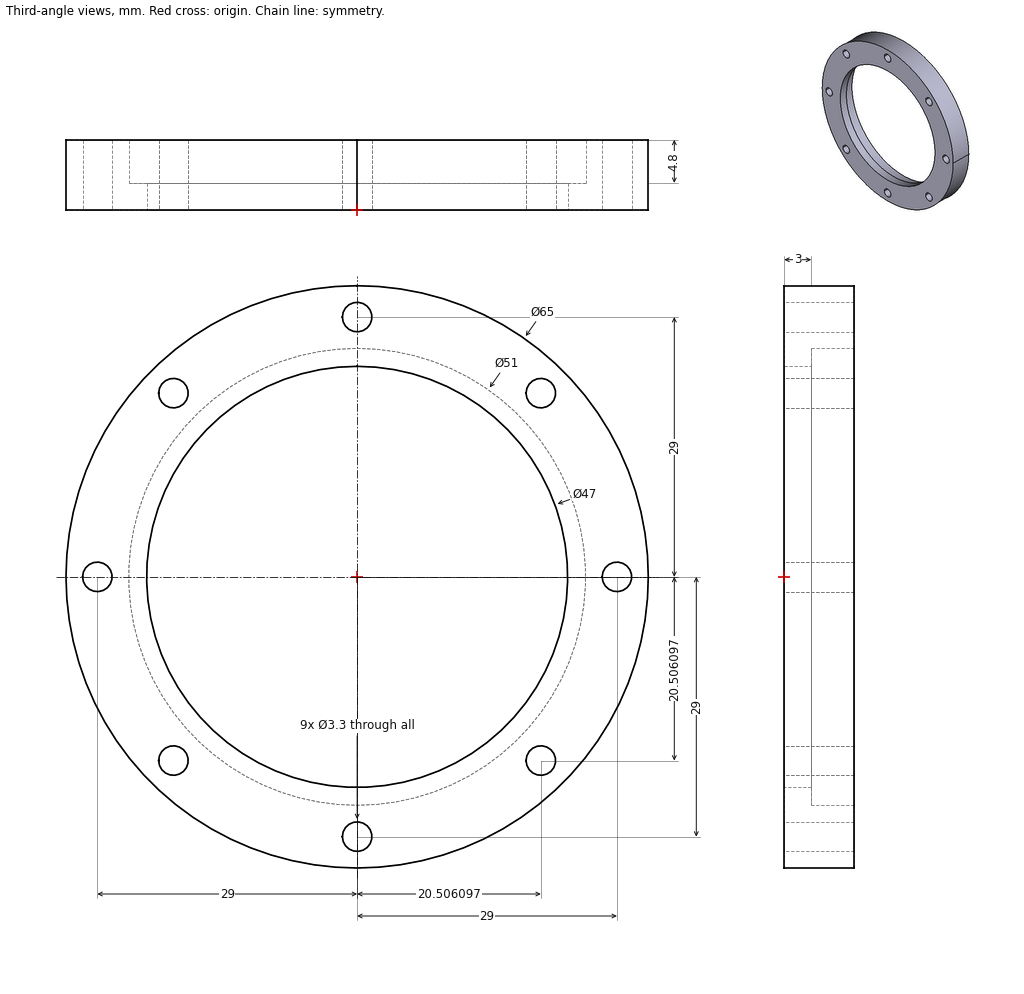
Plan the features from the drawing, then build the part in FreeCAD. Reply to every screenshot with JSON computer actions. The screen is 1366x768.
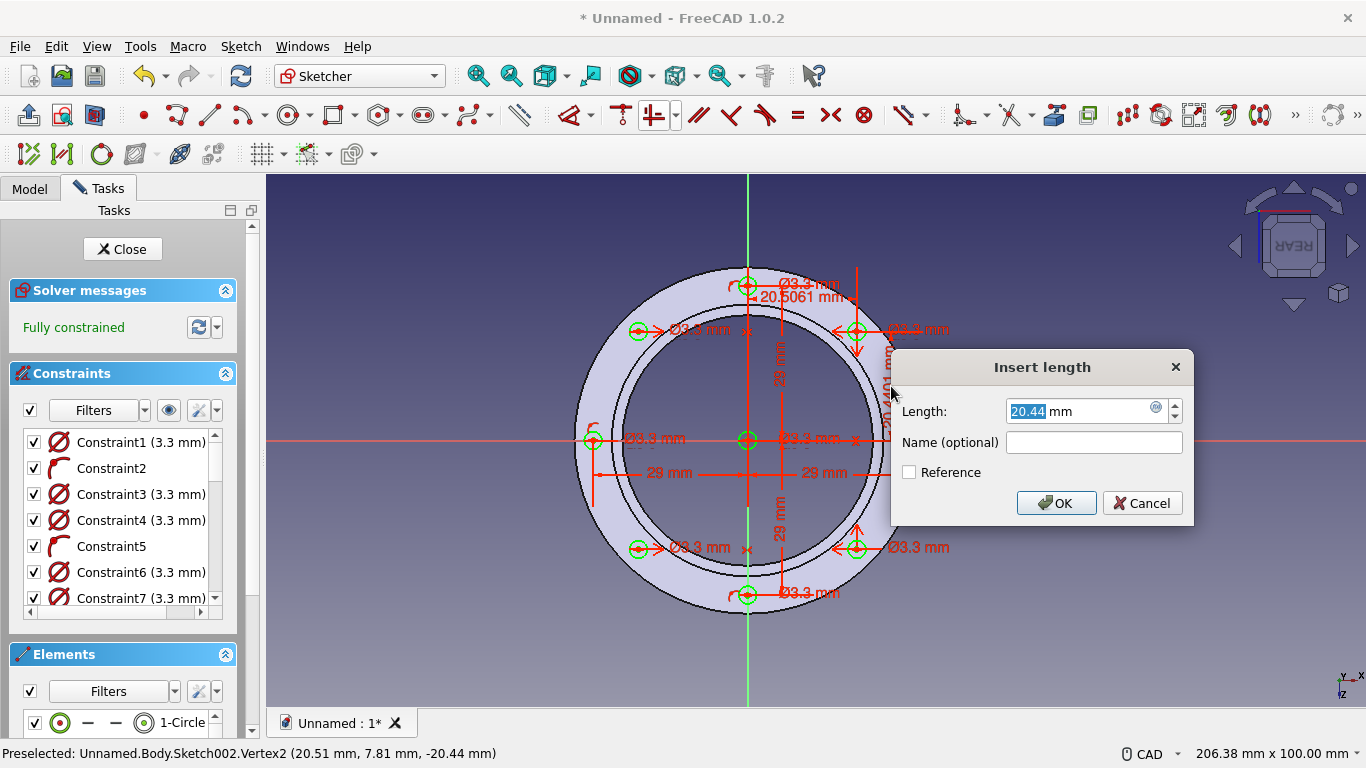
{"action": "type", "text": "20.506097"}
{"action": "key", "text": "Return"}
{"action": "key", "text": "Escape"}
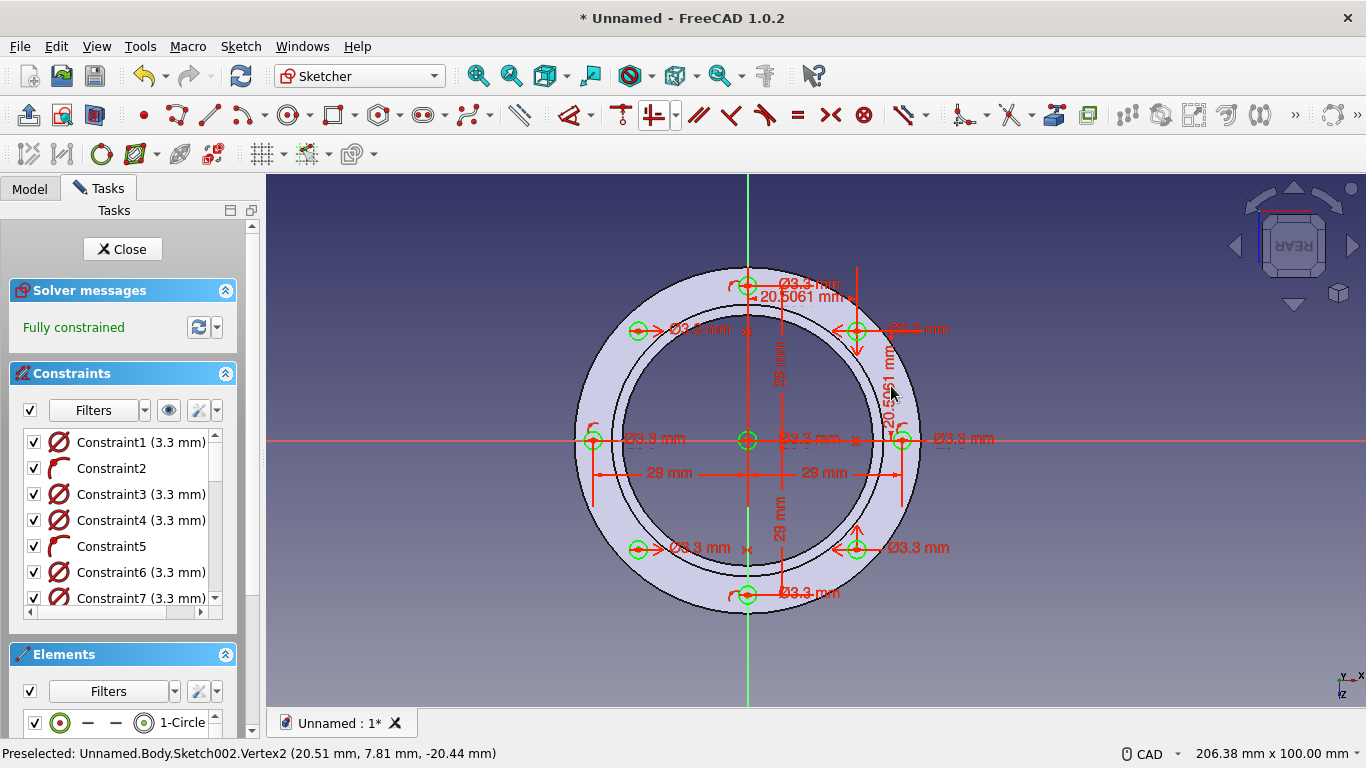
{"action": "left_click", "coordinate": [123, 249]}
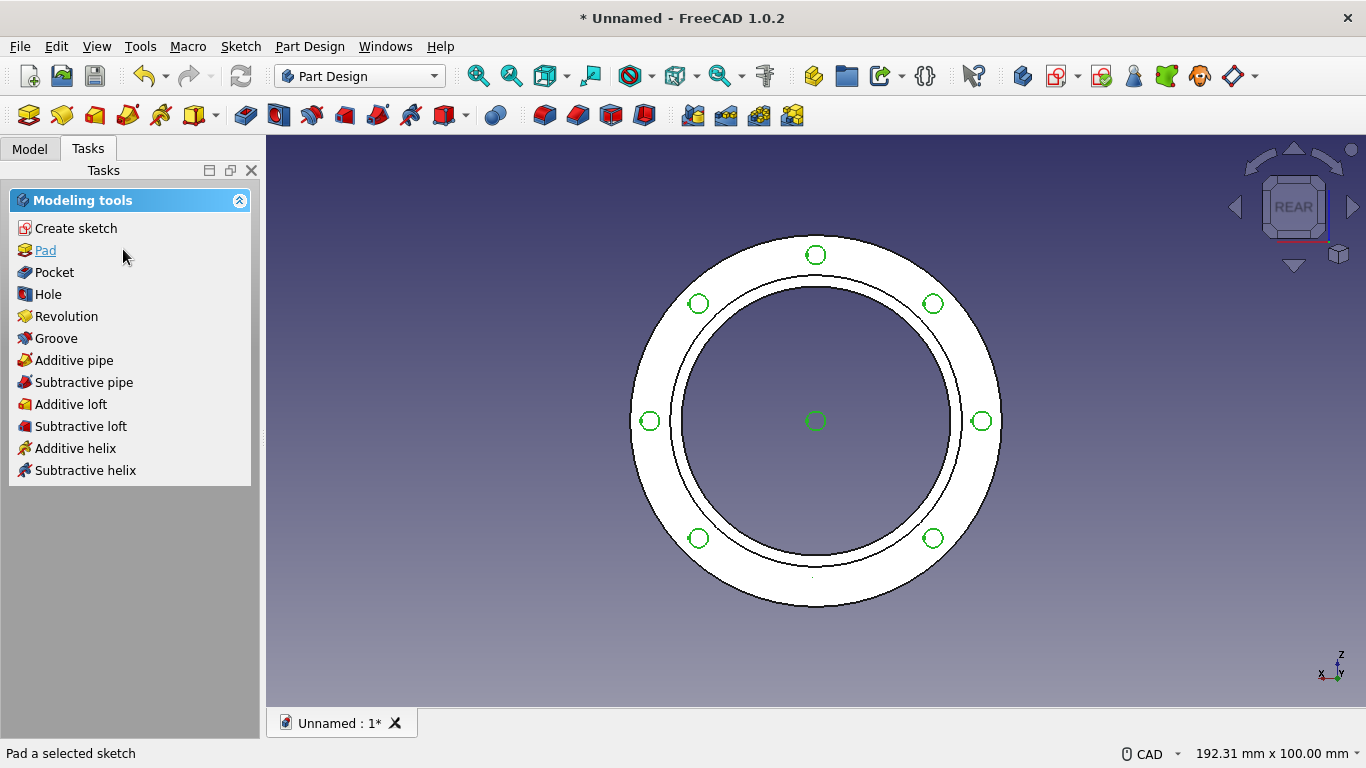
{"action": "left_click", "coordinate": [279, 116]}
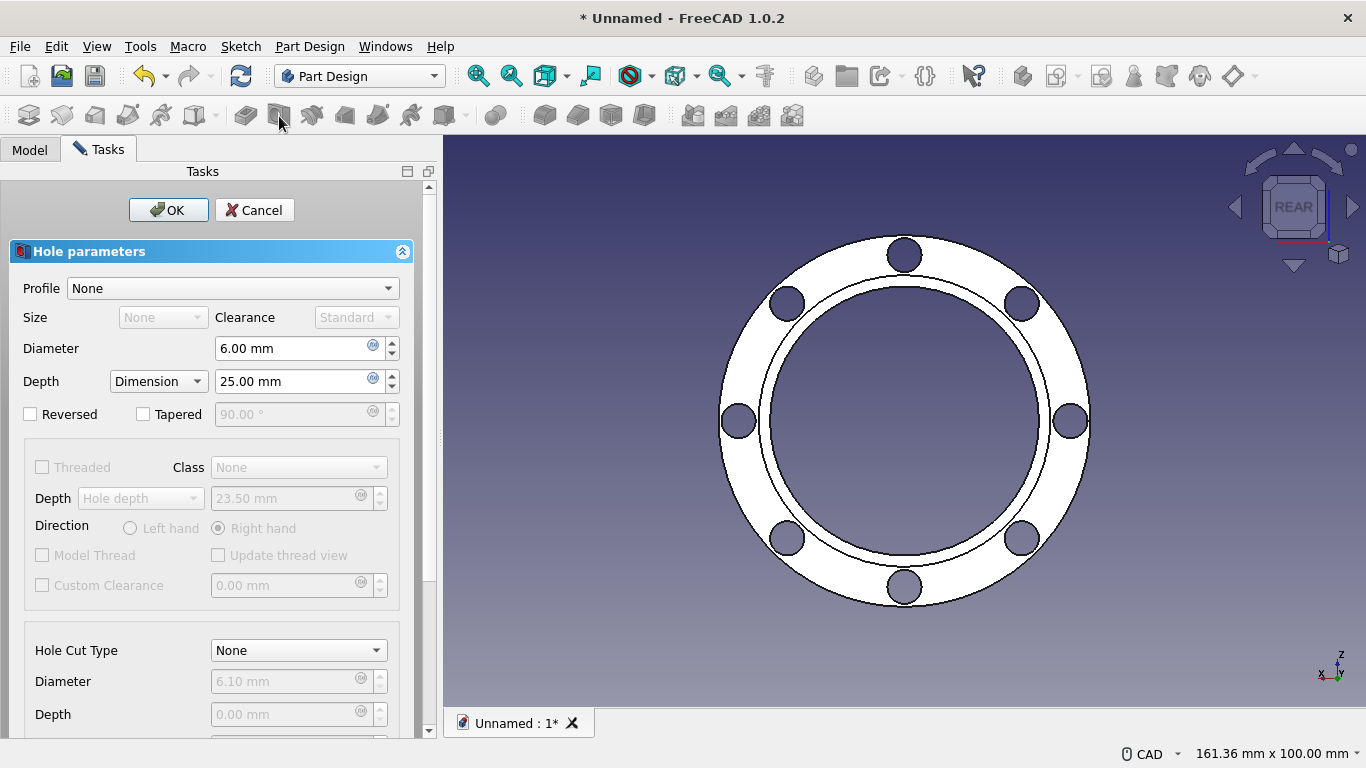
{"action": "triple_click", "coordinate": [300, 348]}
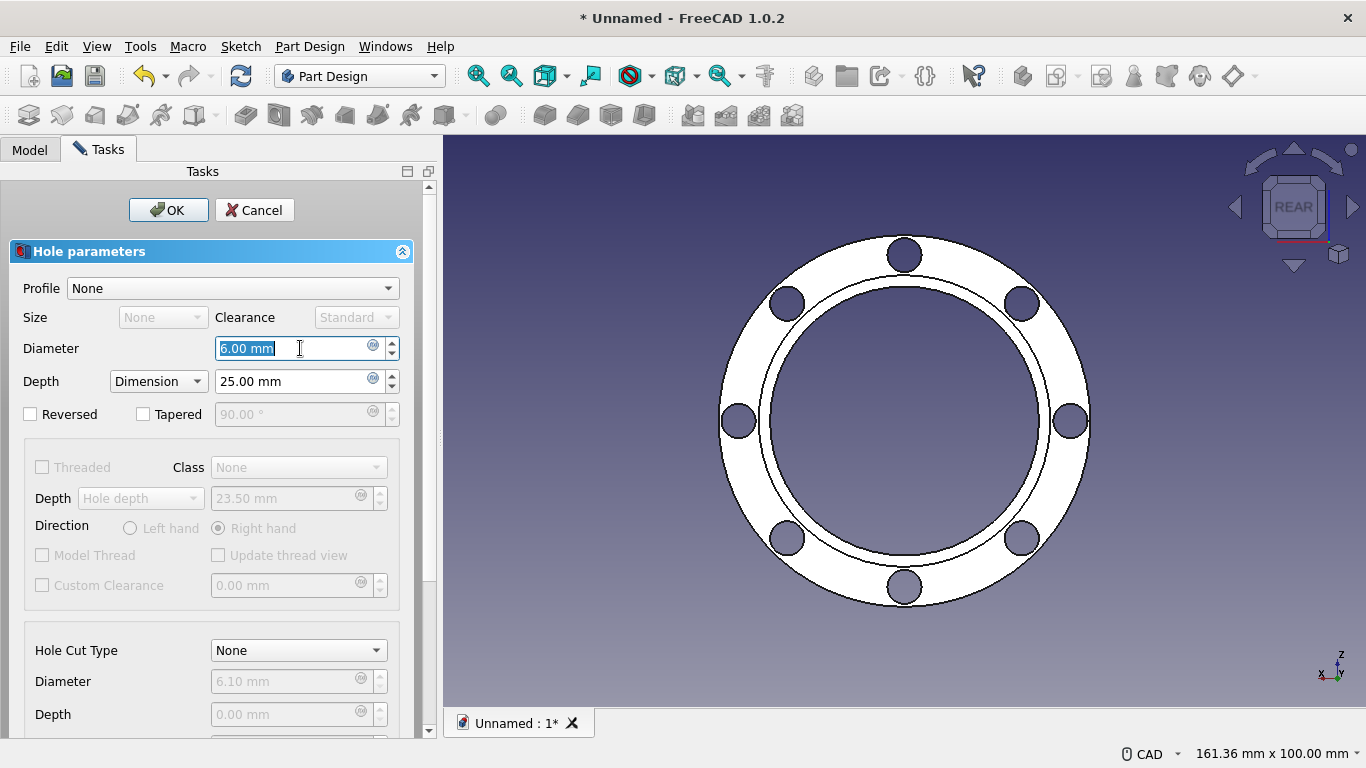
{"action": "type", "text": "3.3"}
{"action": "key", "text": "Tab"}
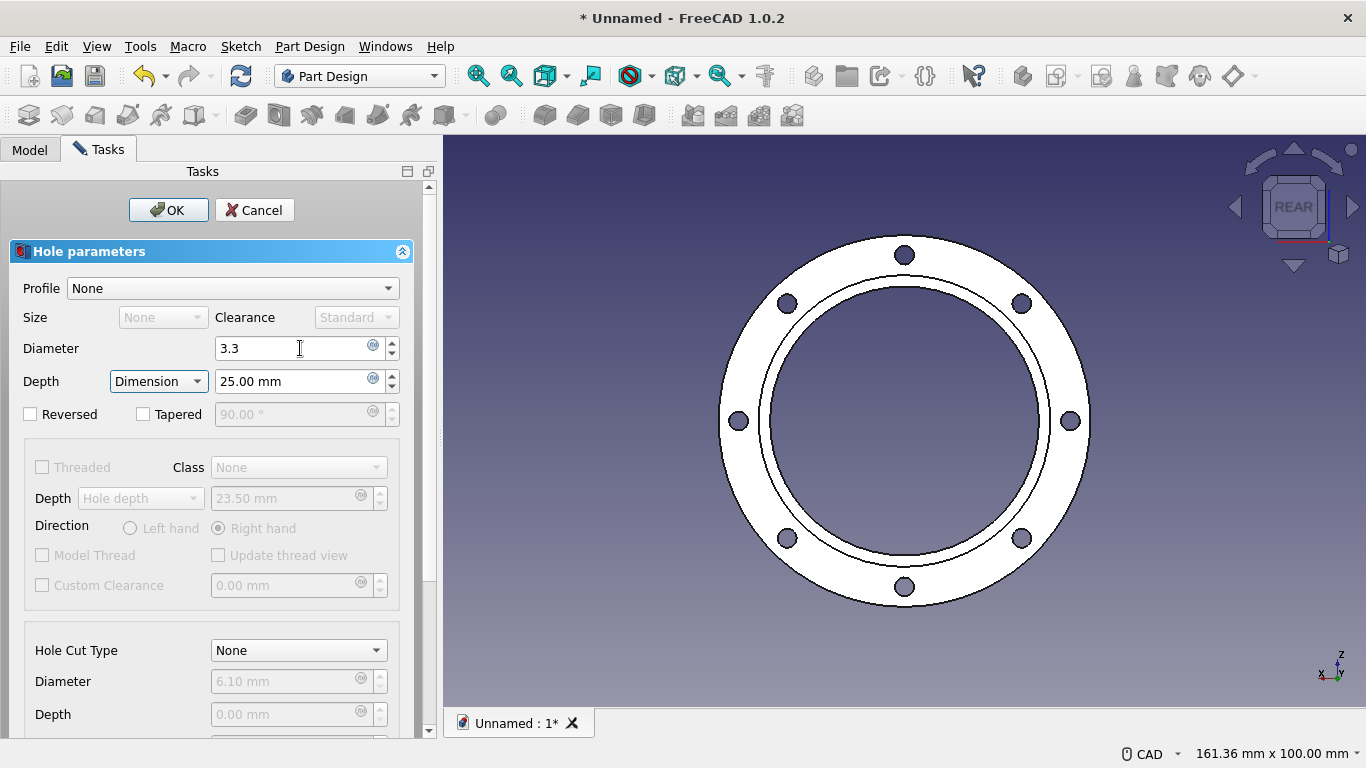
{"action": "left_click", "coordinate": [160, 382]}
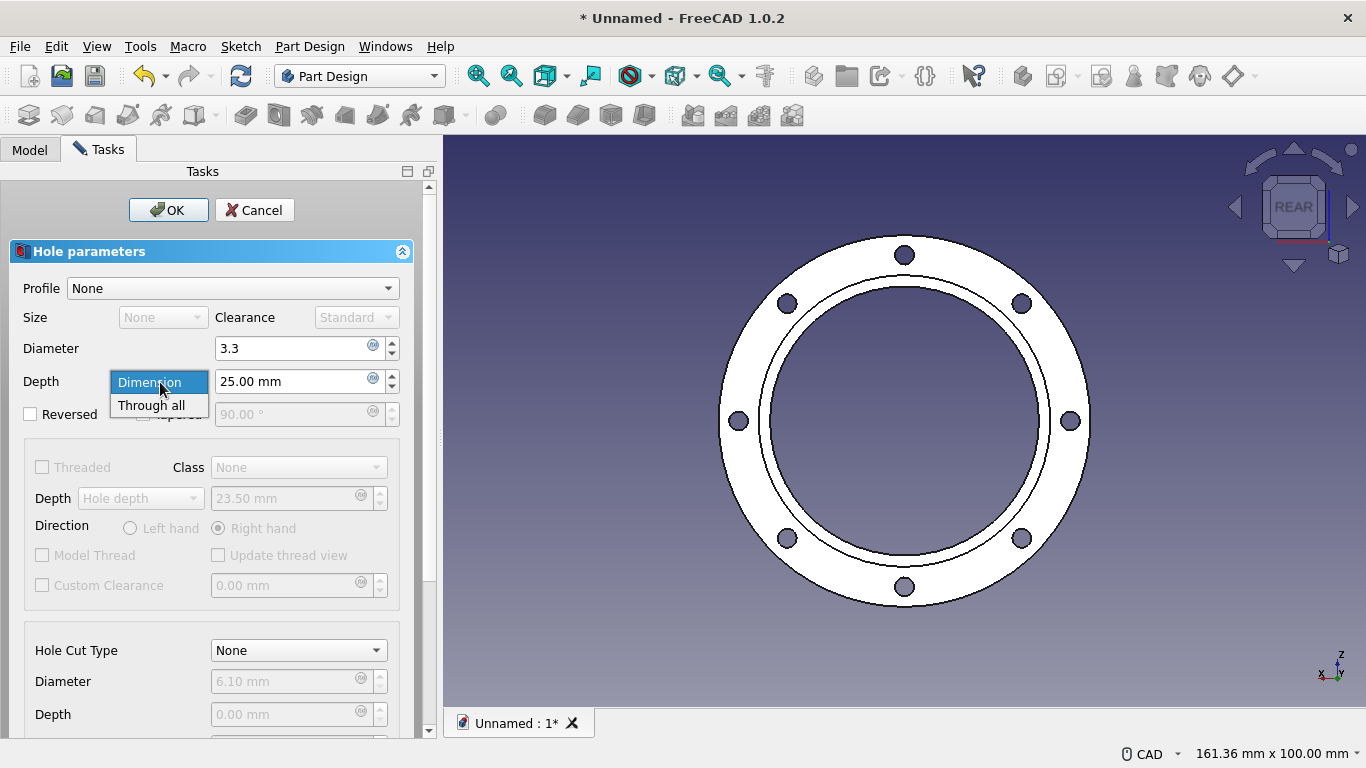
{"action": "left_click", "coordinate": [158, 406]}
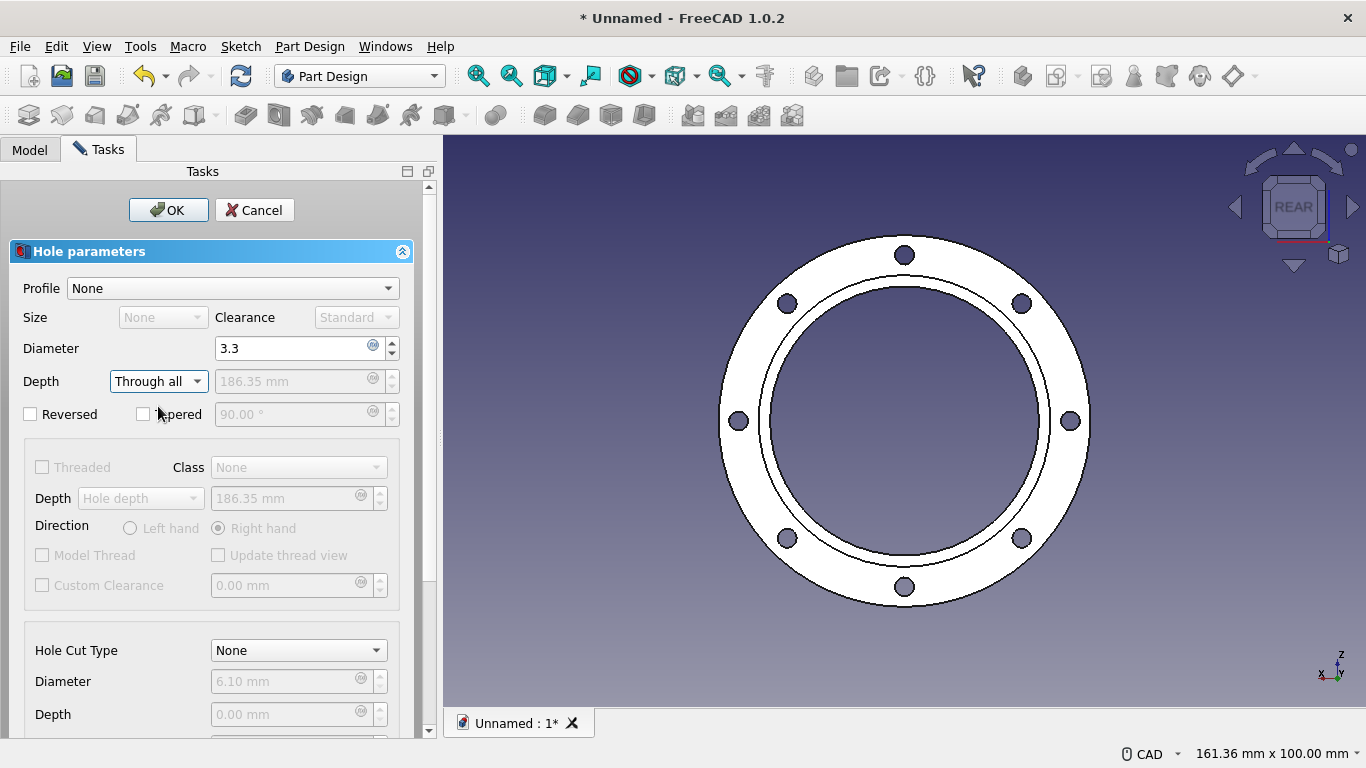
{"action": "left_click", "coordinate": [169, 210]}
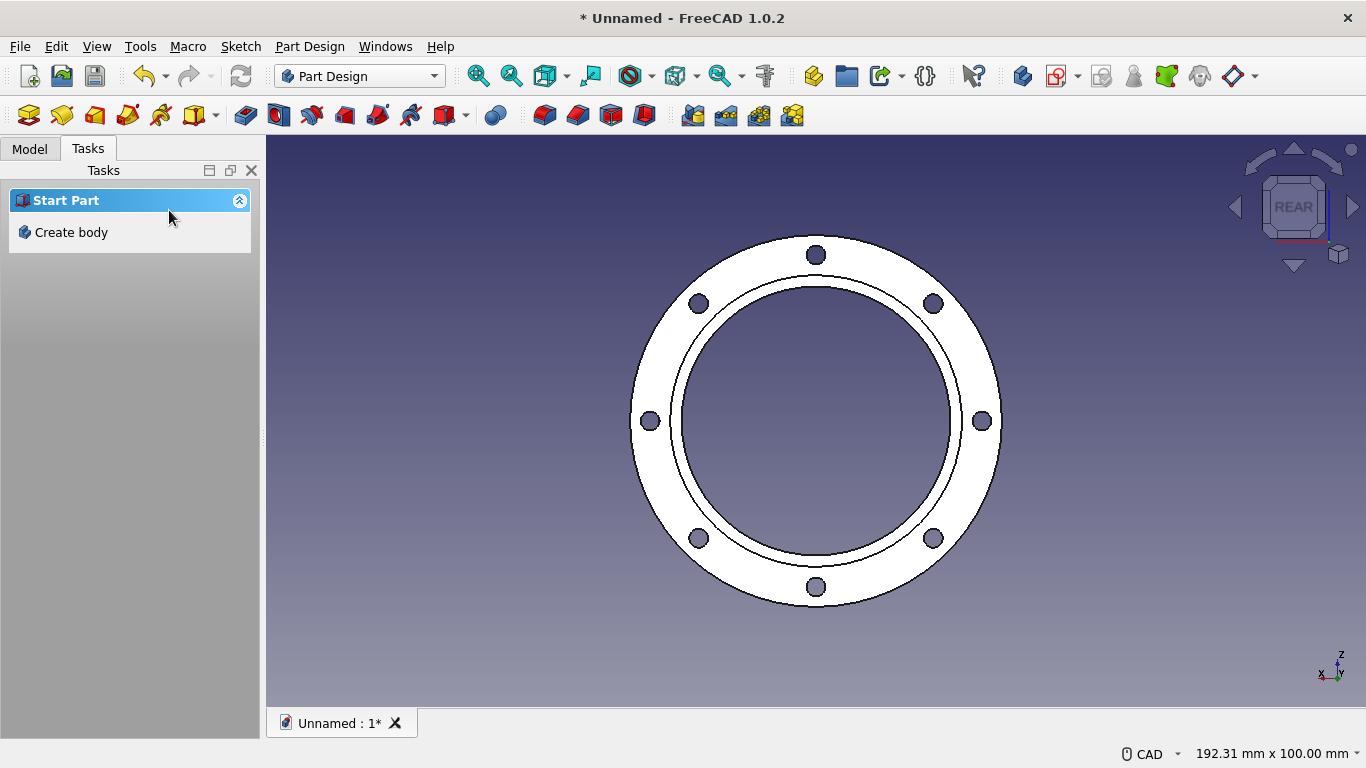
{"action": "key", "text": "0"}